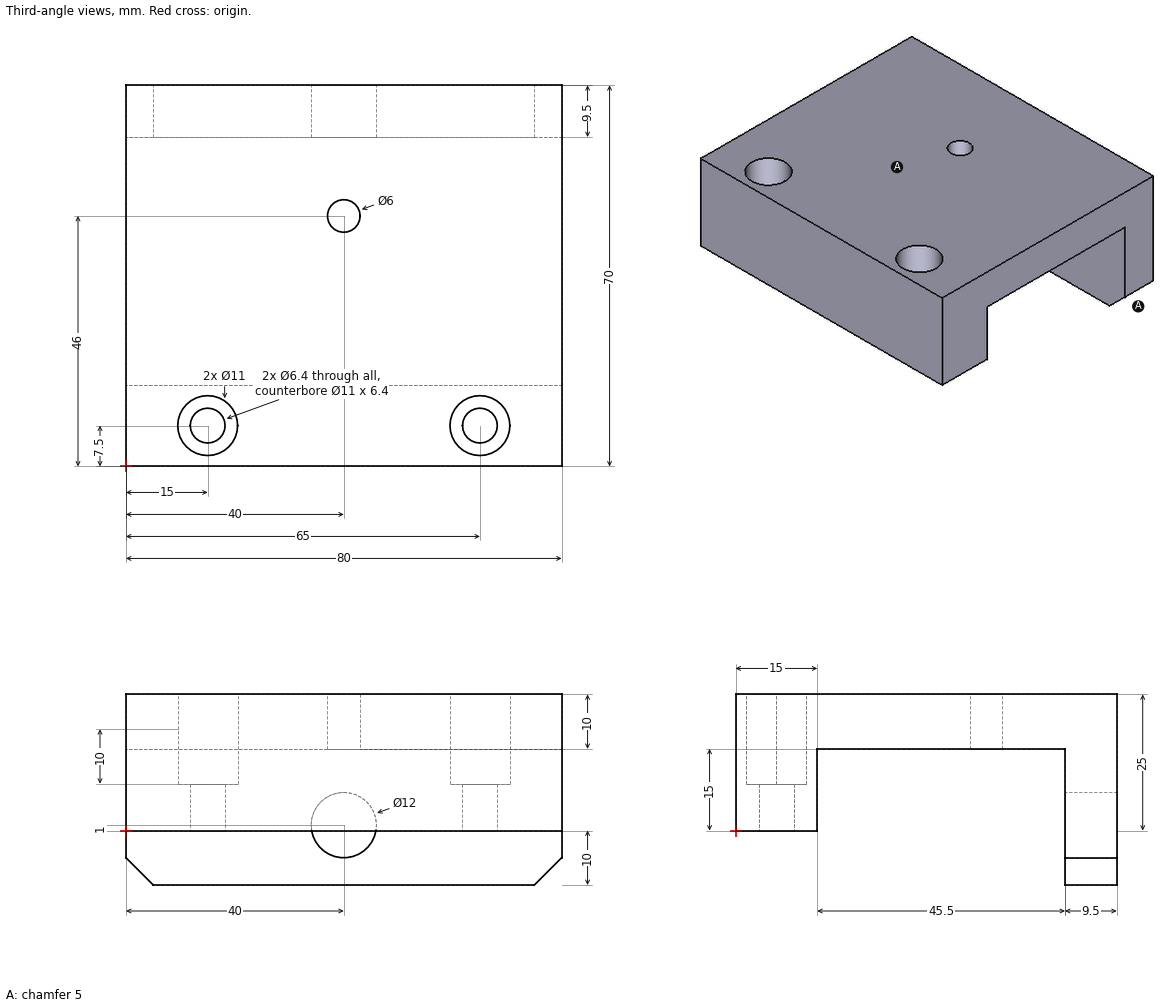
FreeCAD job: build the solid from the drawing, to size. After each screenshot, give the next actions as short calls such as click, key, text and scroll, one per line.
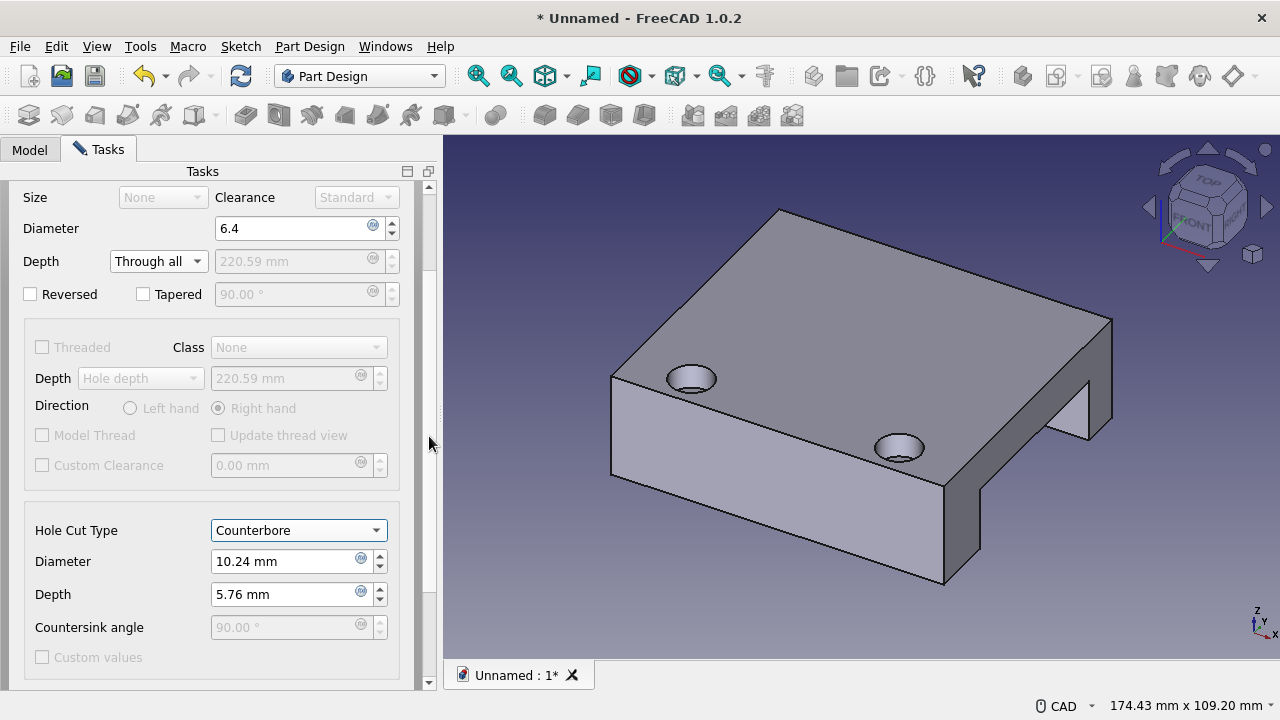
triple_click(292, 562)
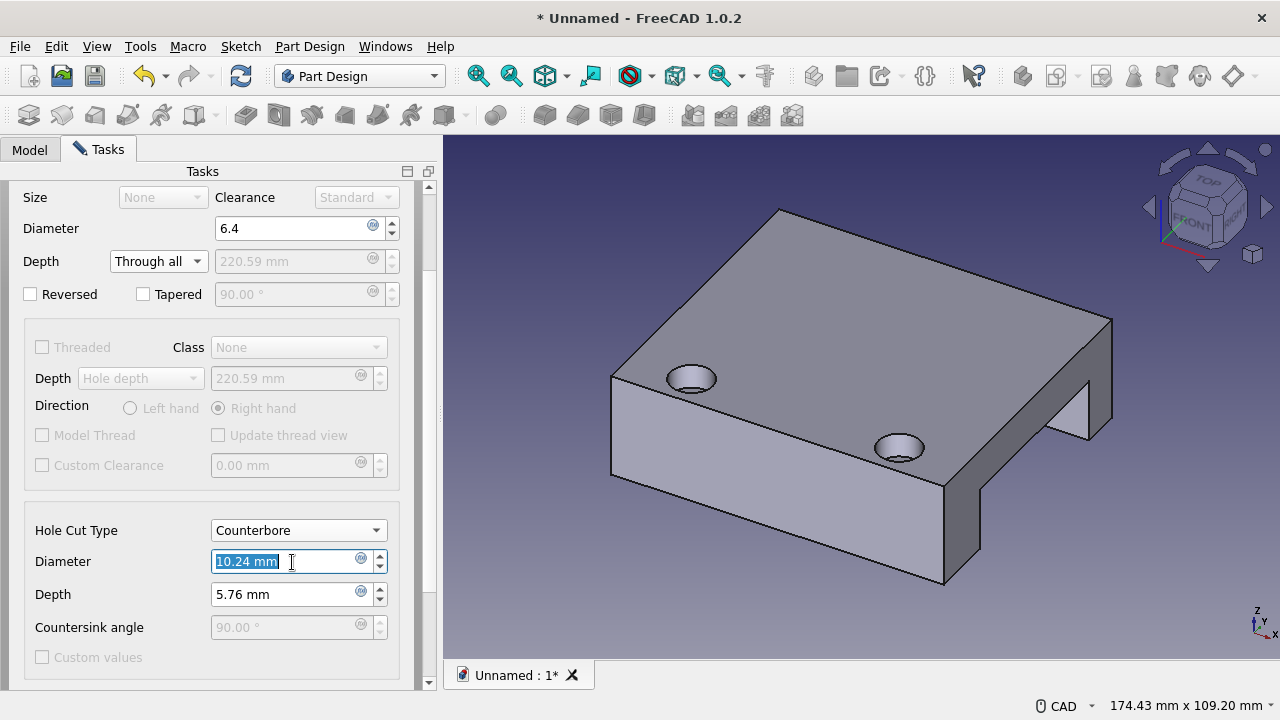
text(11)
key(Tab)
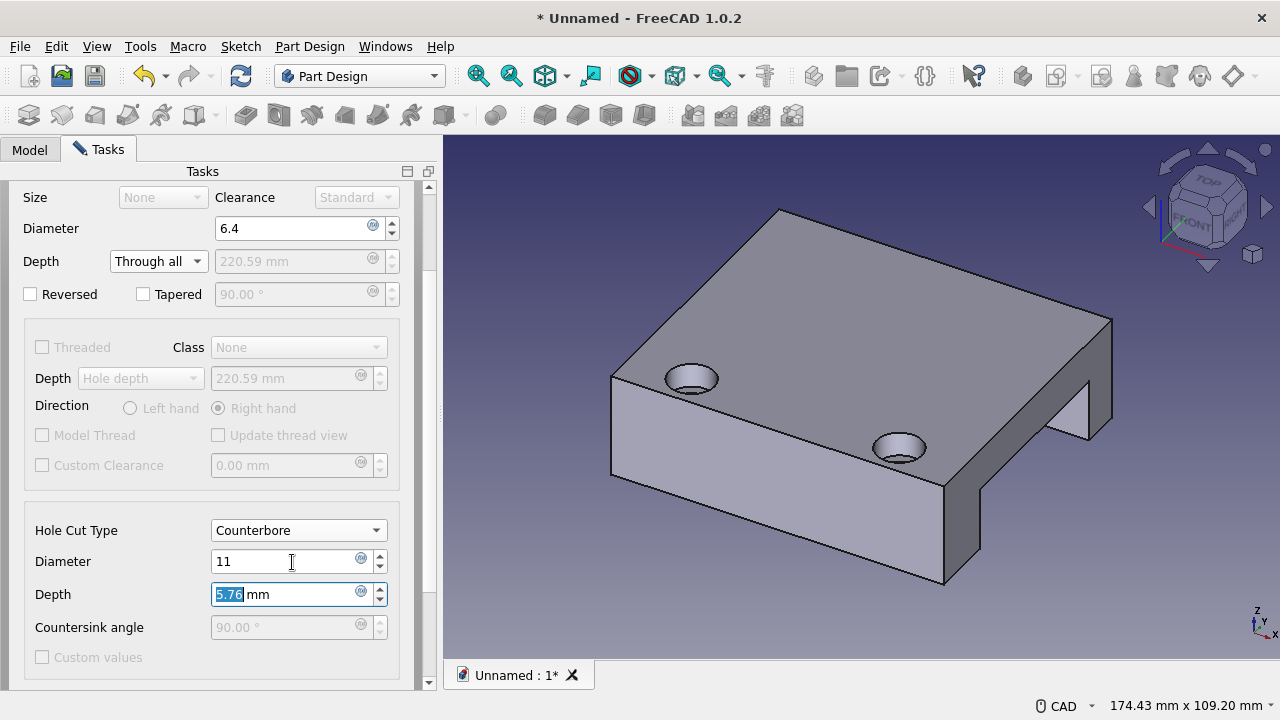
text(6.4)
key(Tab)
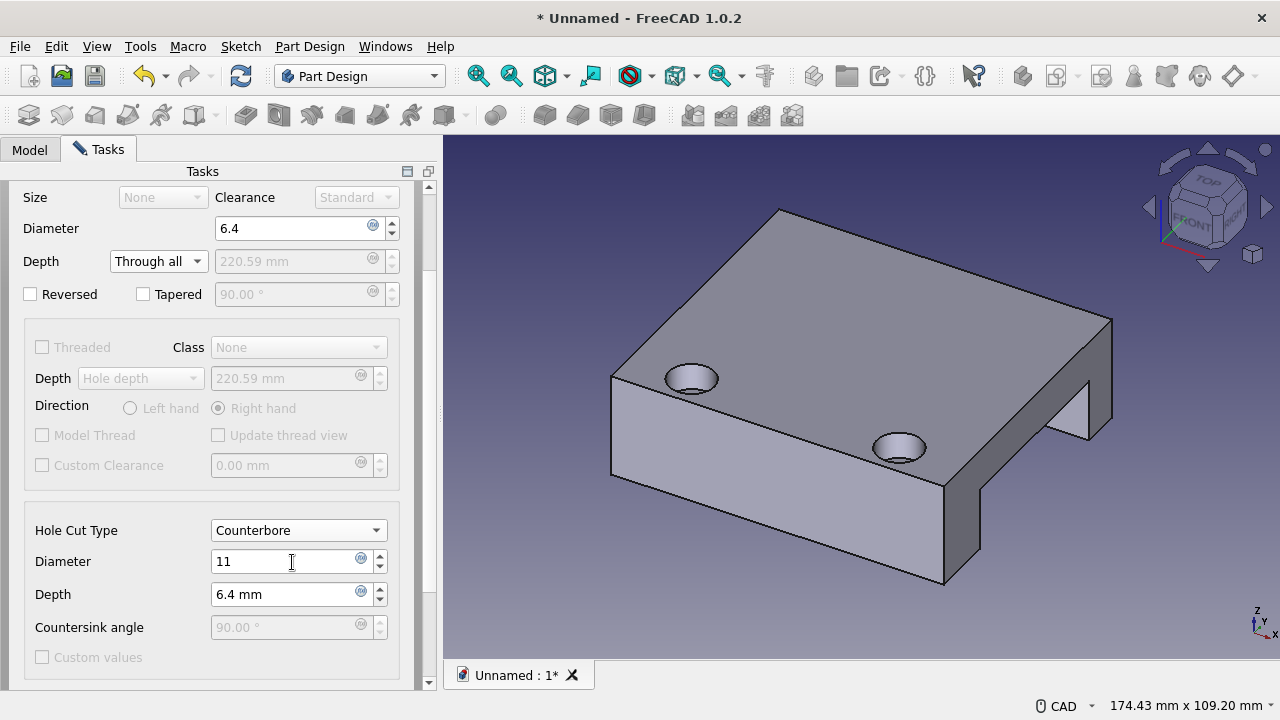
scroll(429, 436, up, 3)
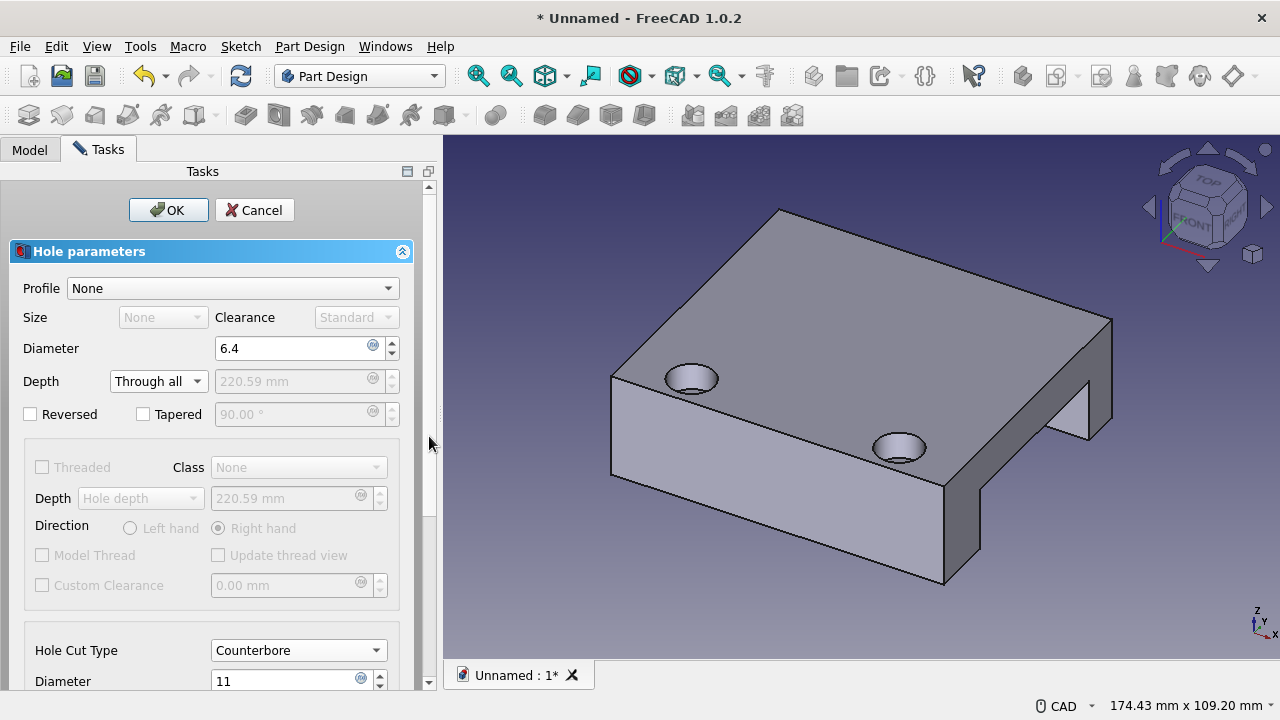
click(169, 210)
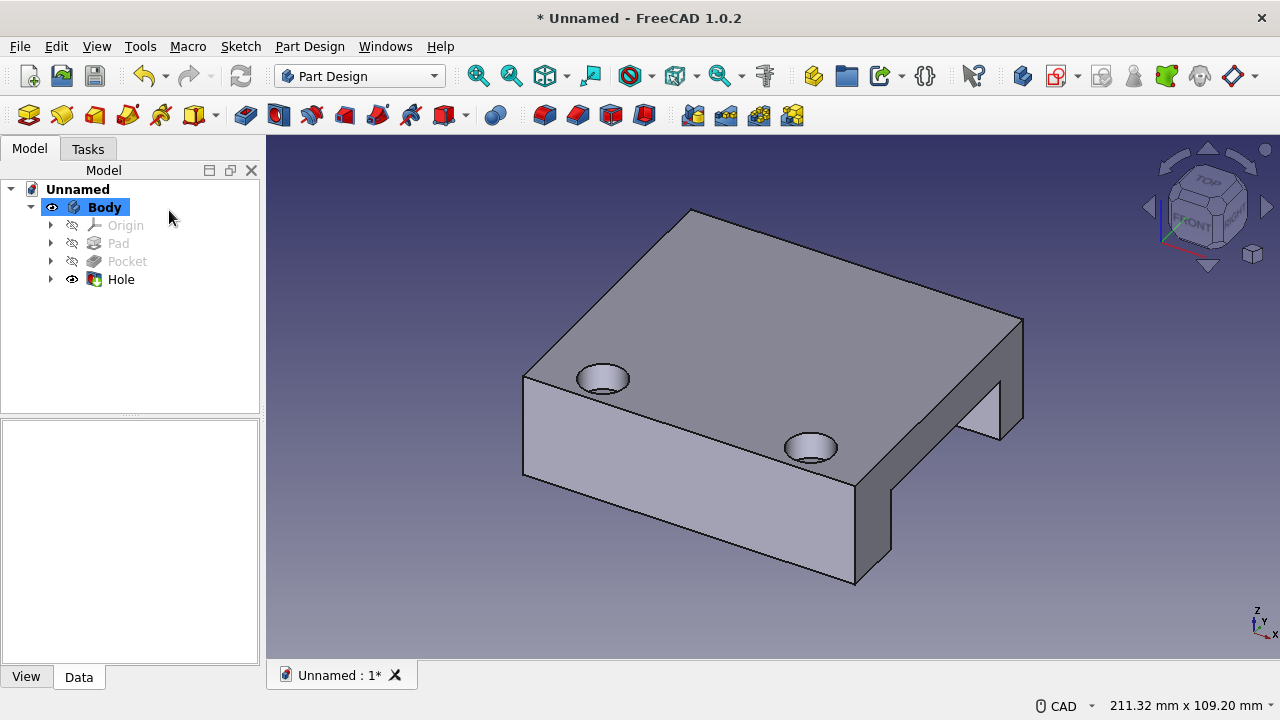
scroll(816, 484, up, 5)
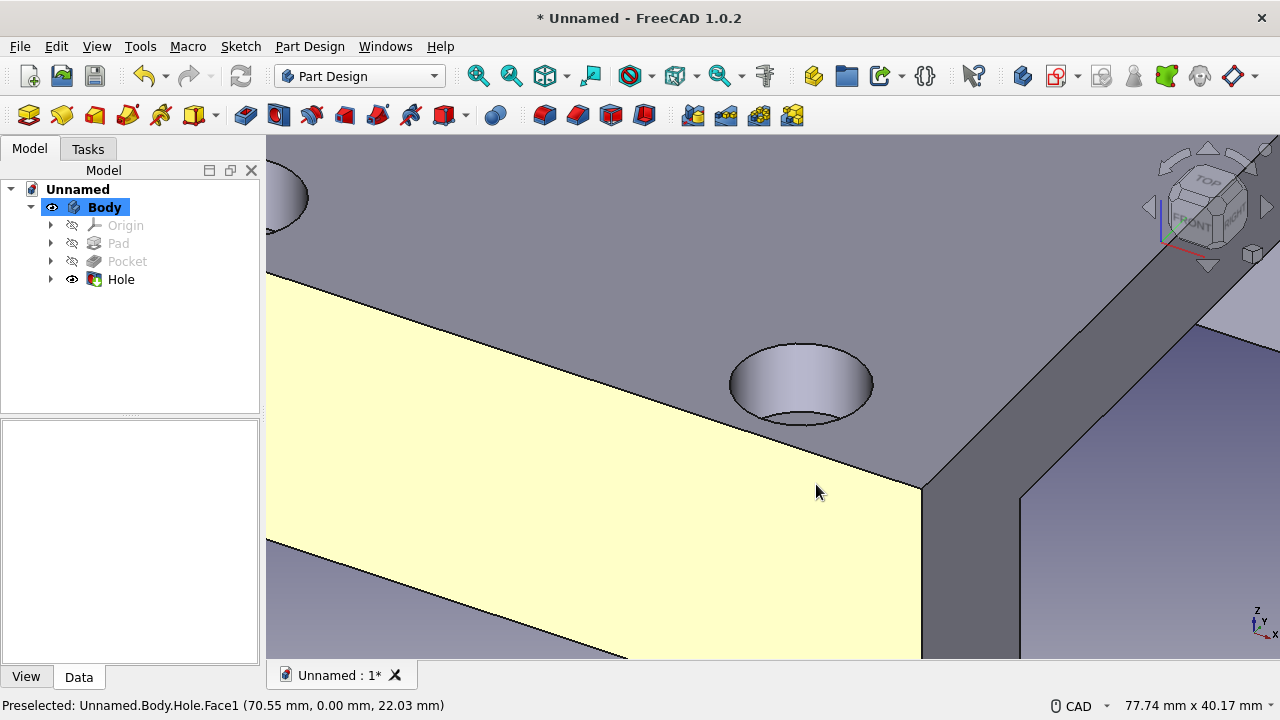
click(479, 76)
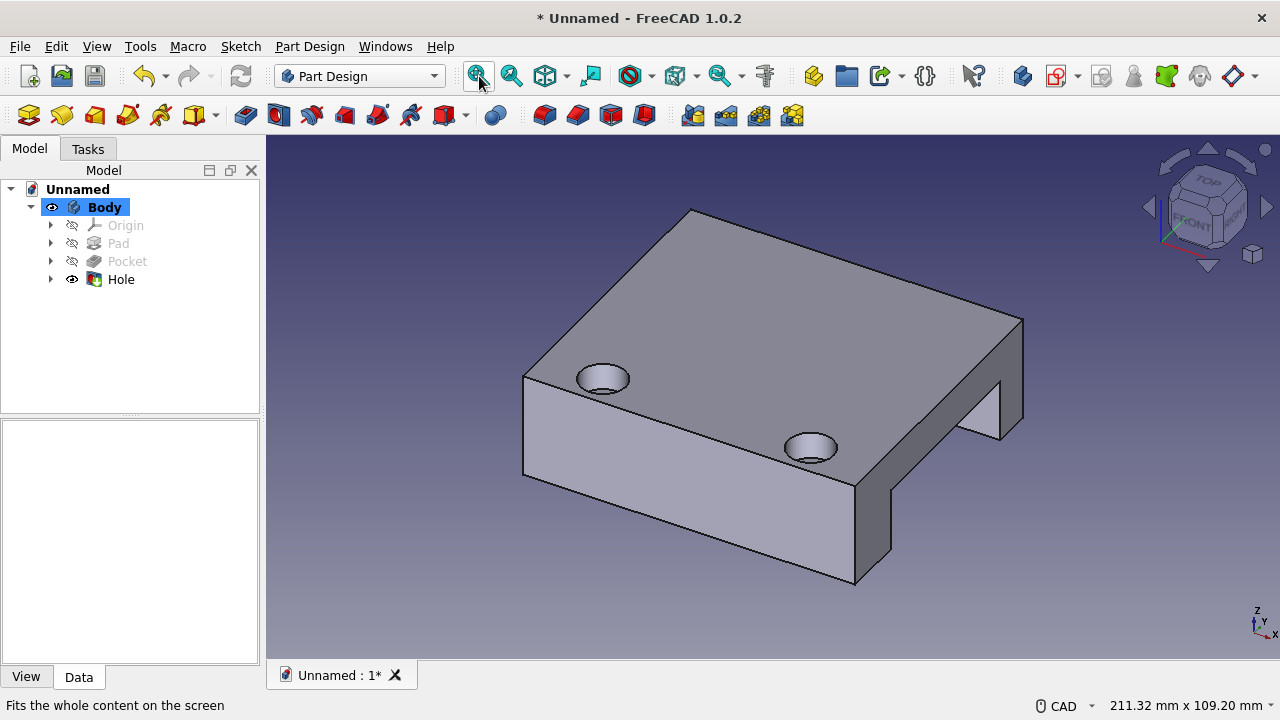
key(0)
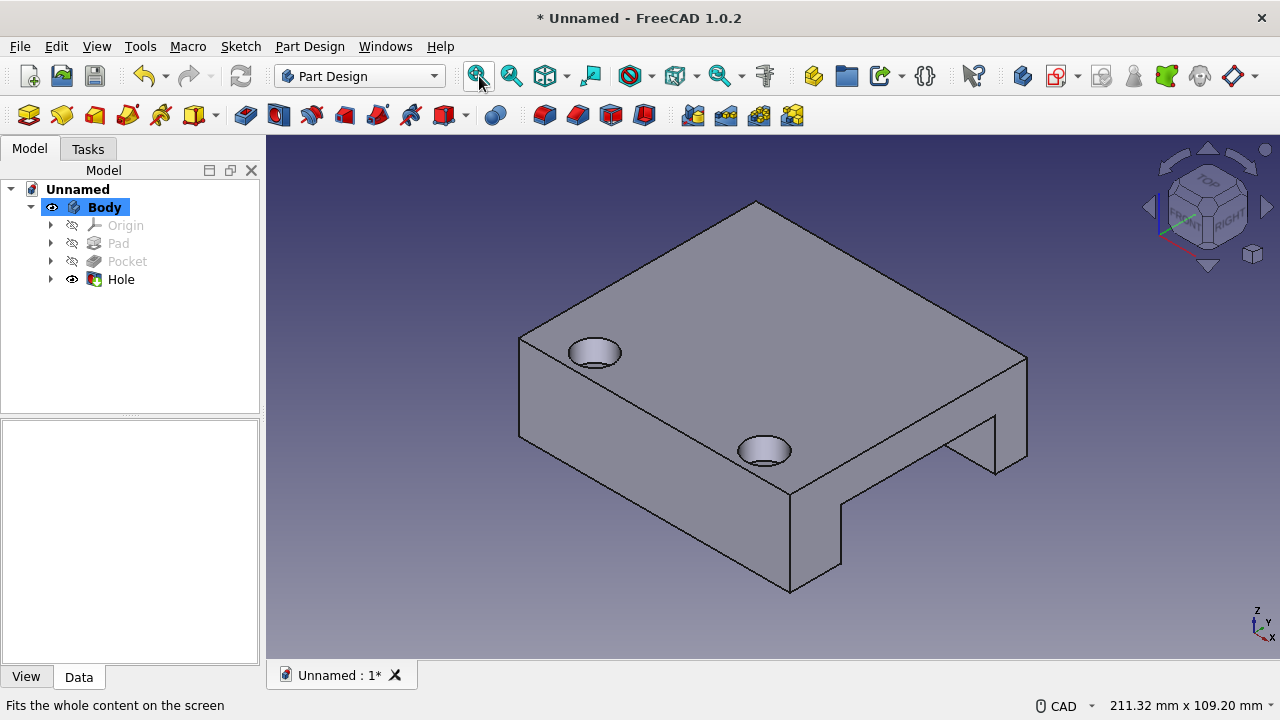
scroll(765, 487, up, 5)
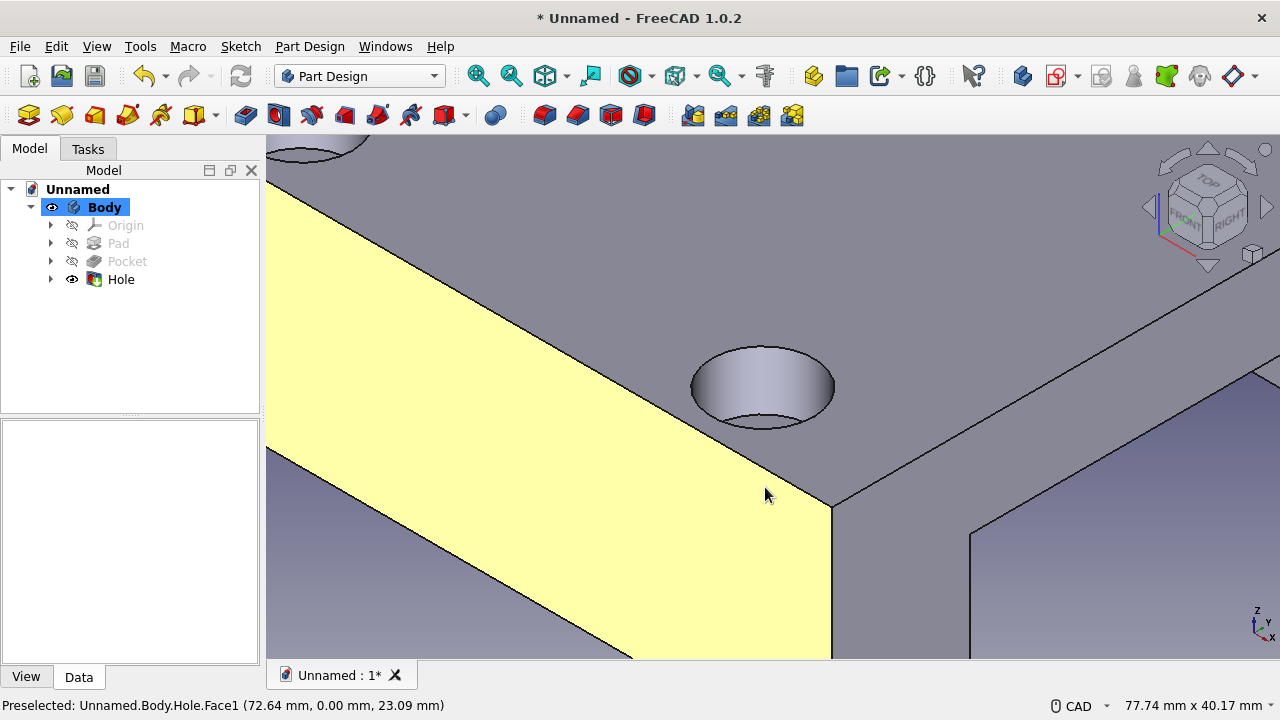
click(479, 76)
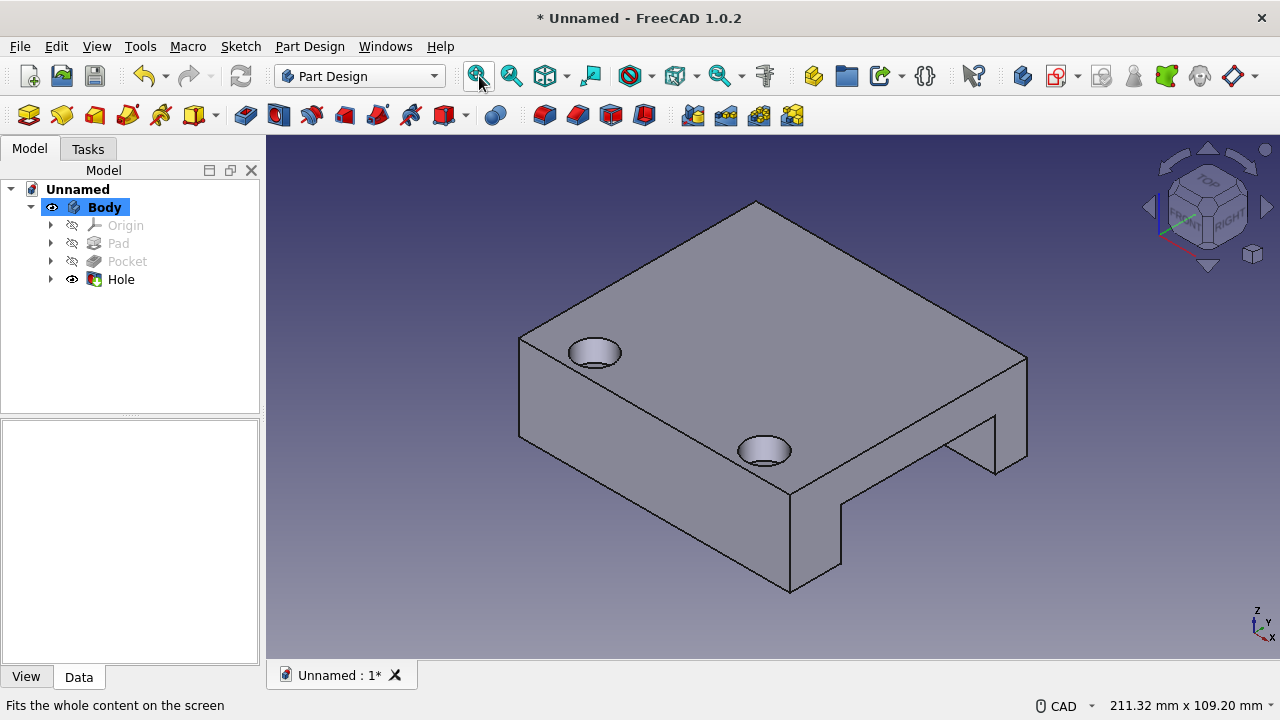
key(2)